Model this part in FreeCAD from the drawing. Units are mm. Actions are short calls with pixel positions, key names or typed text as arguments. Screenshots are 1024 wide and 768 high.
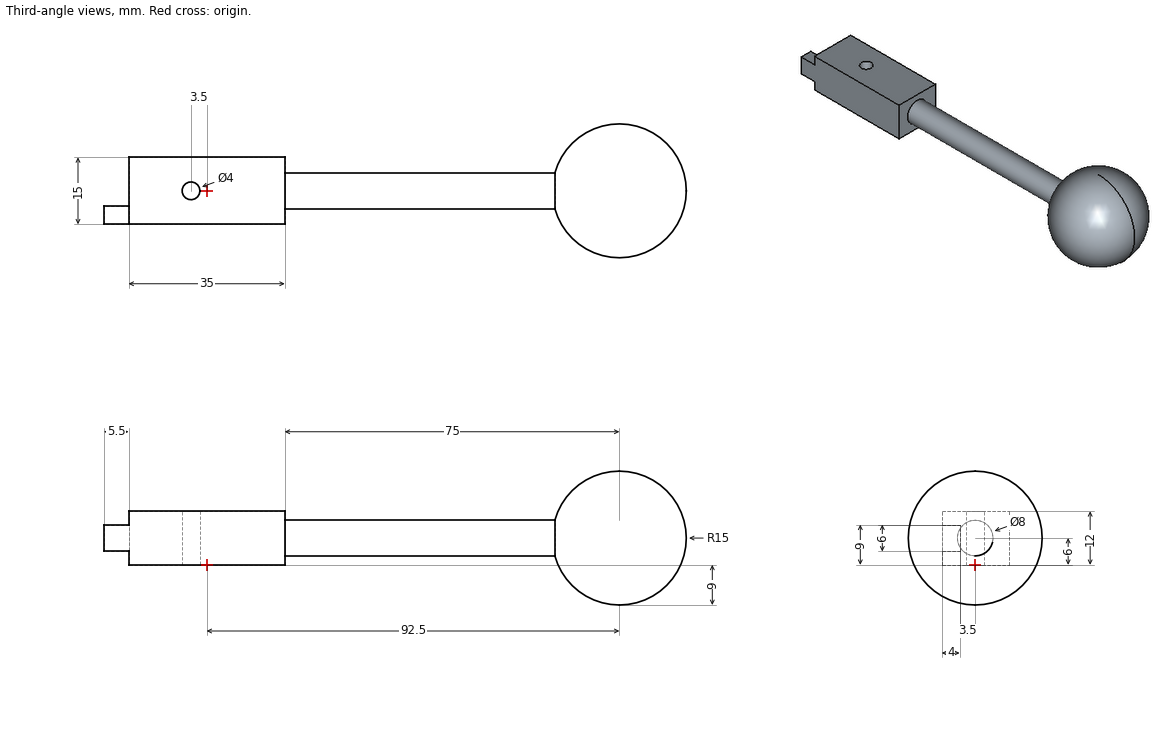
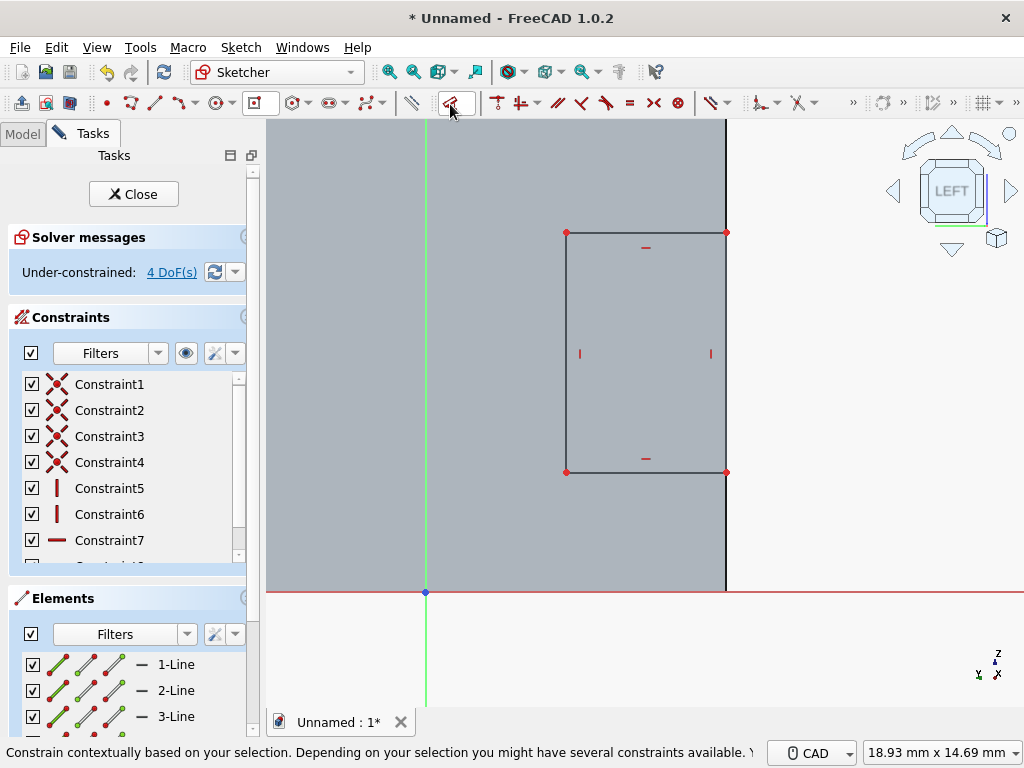
click(566, 305)
click(532, 353)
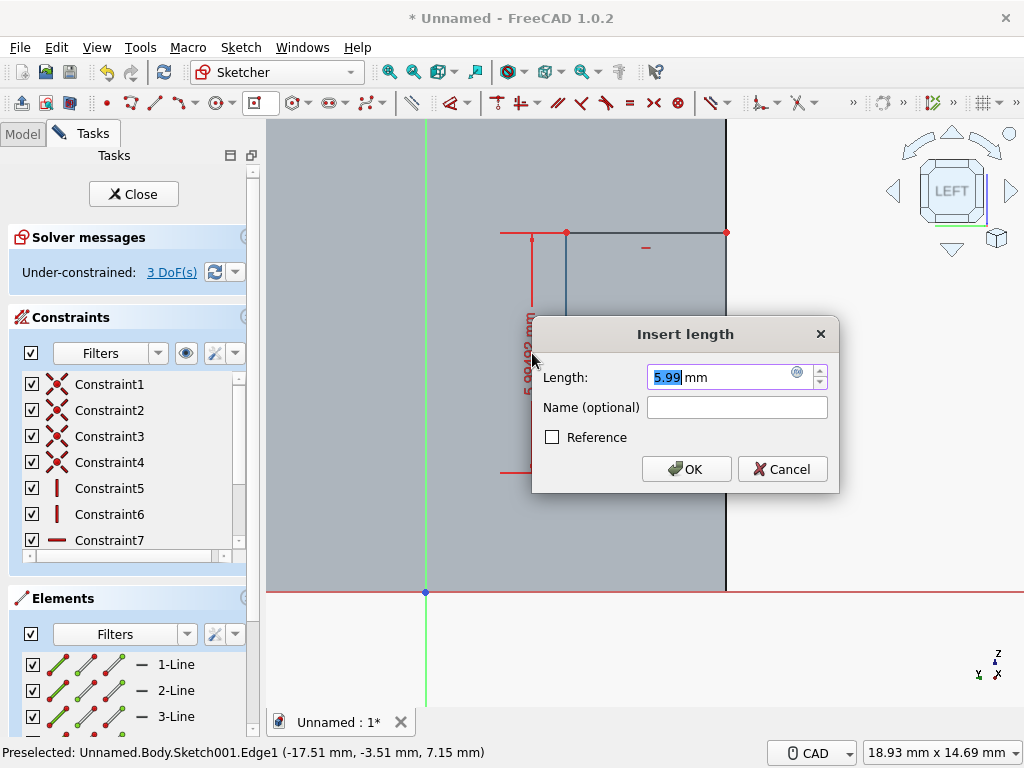
text(6)
key(Return)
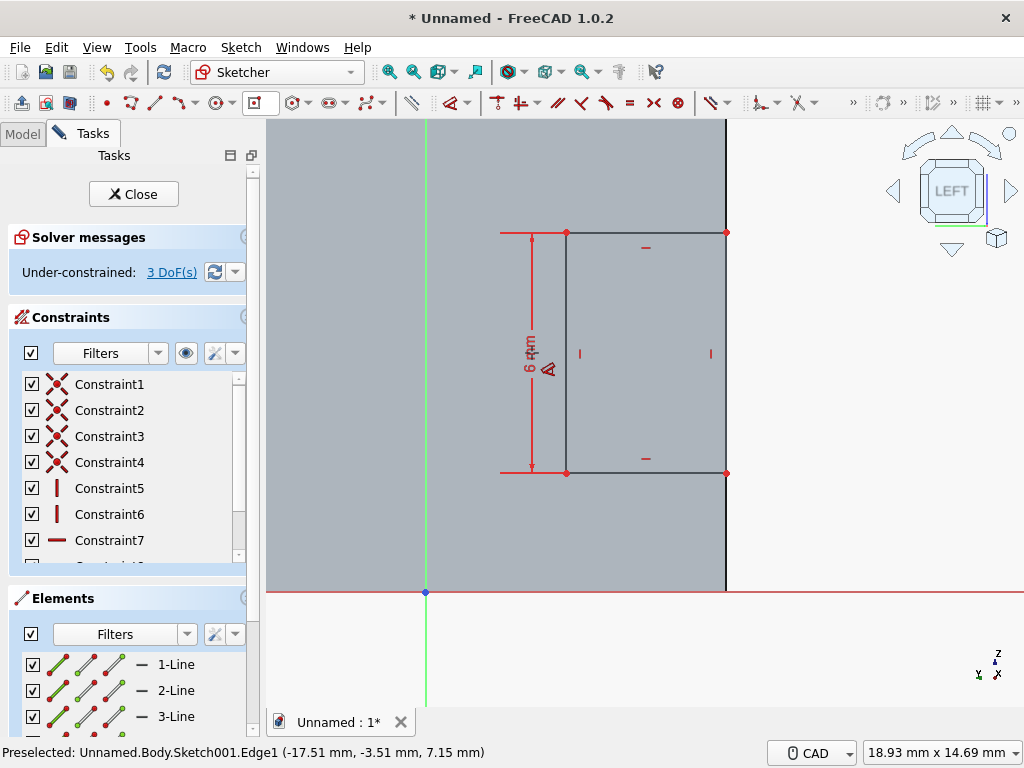
click(614, 473)
click(646, 507)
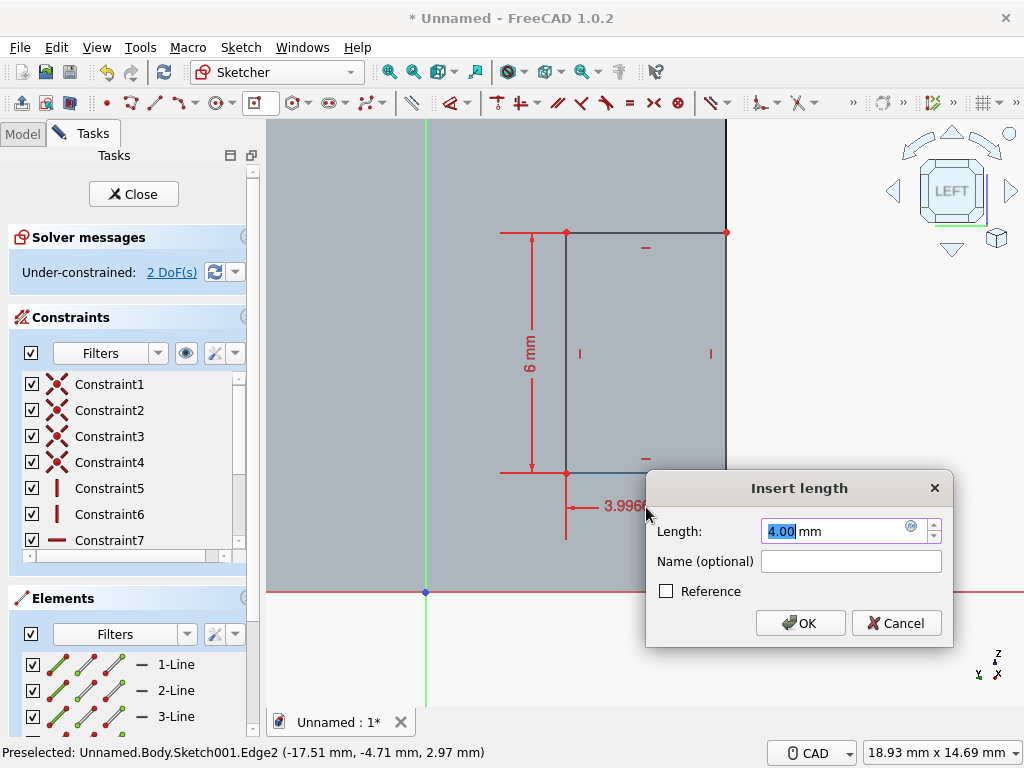
text(4)
key(Return)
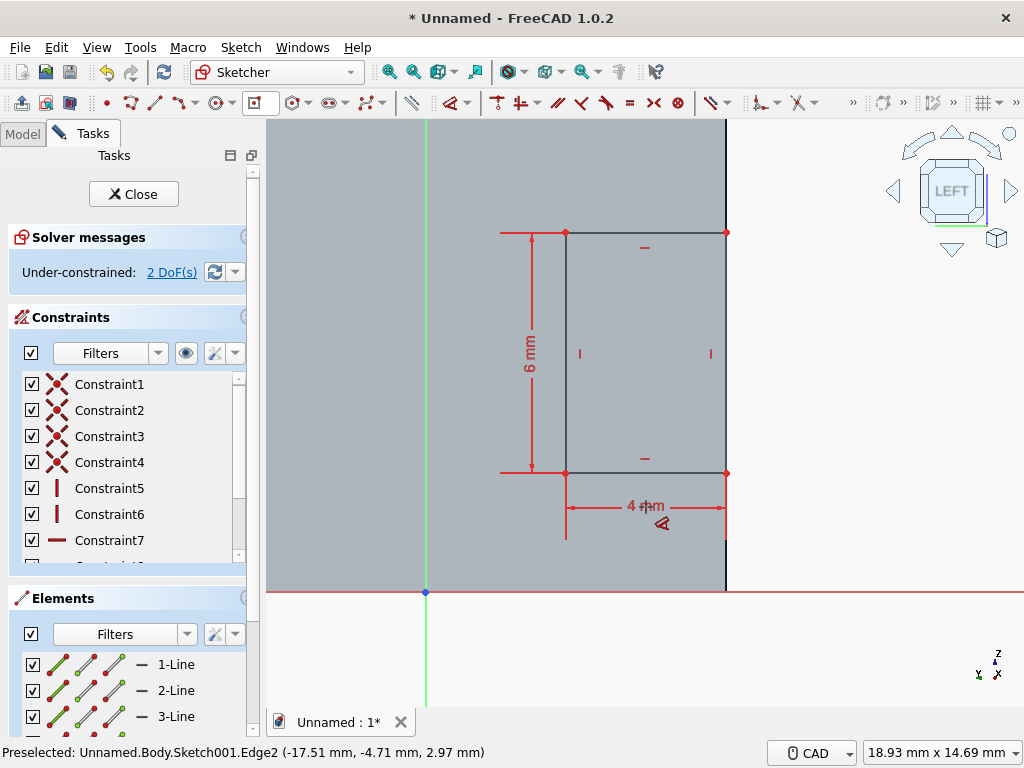
click(566, 233)
click(392, 413)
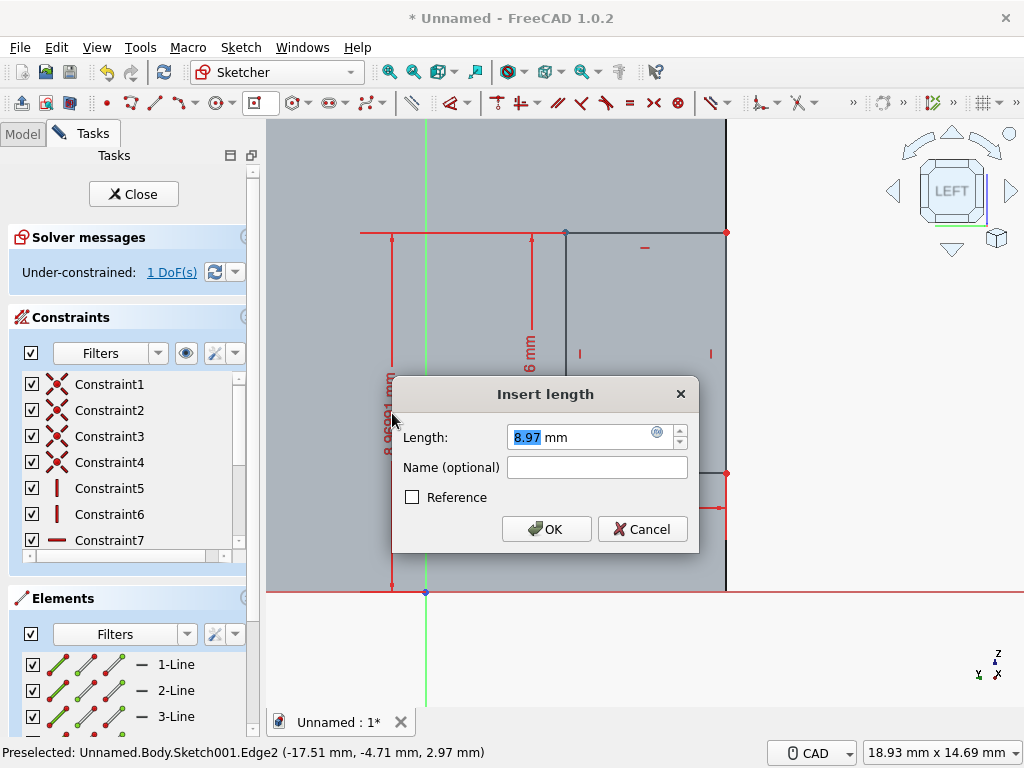
text(9)
key(Return)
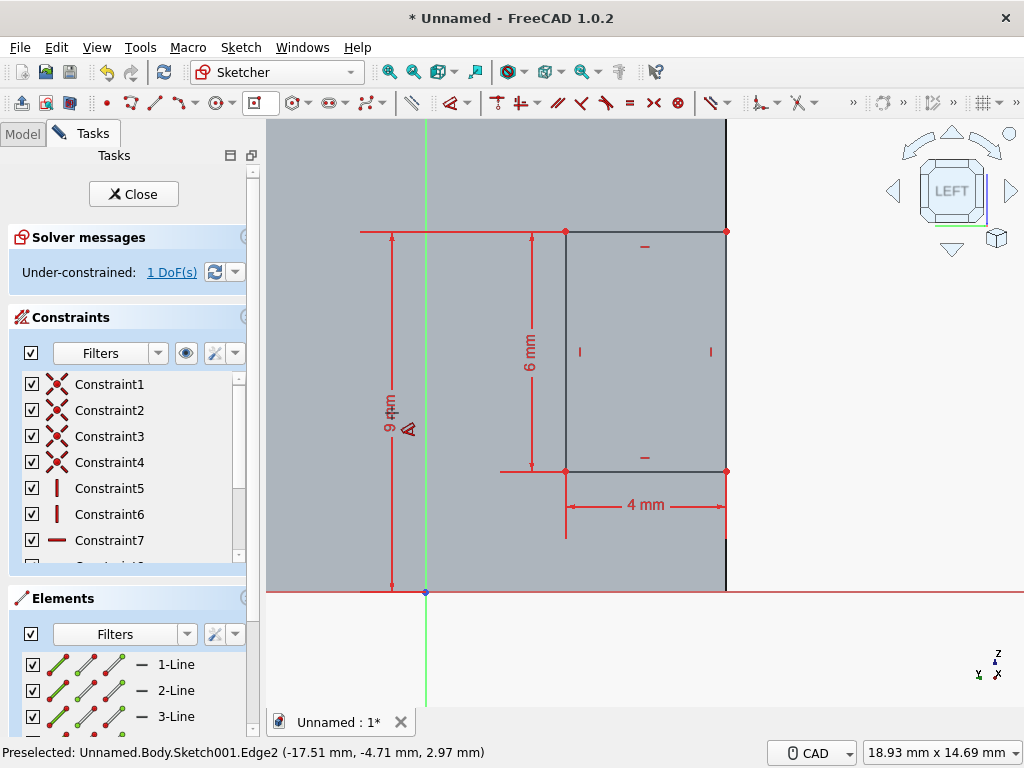
click(566, 232)
click(496, 626)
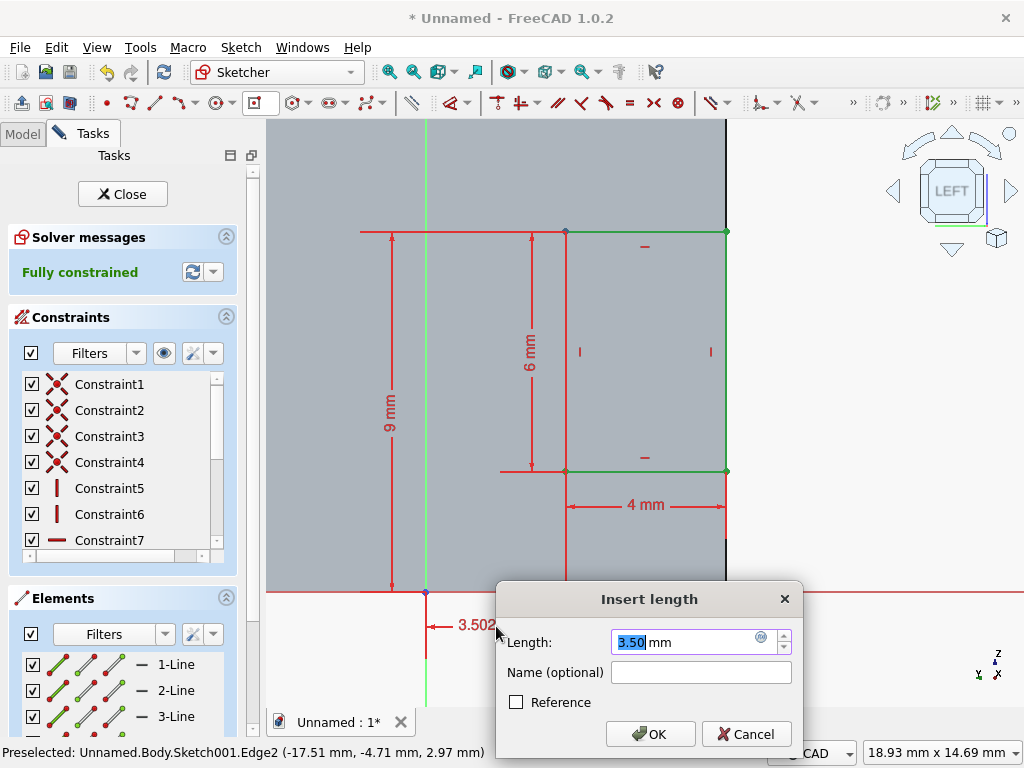
text(3.5)
key(Return)
key(Escape)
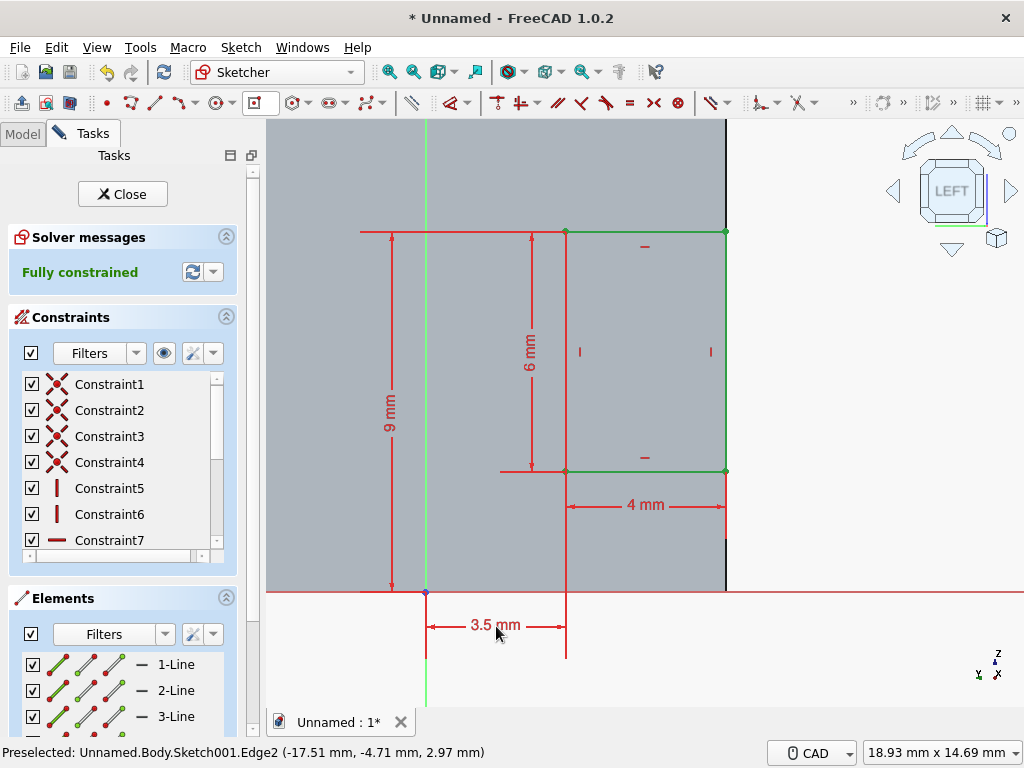
click(123, 194)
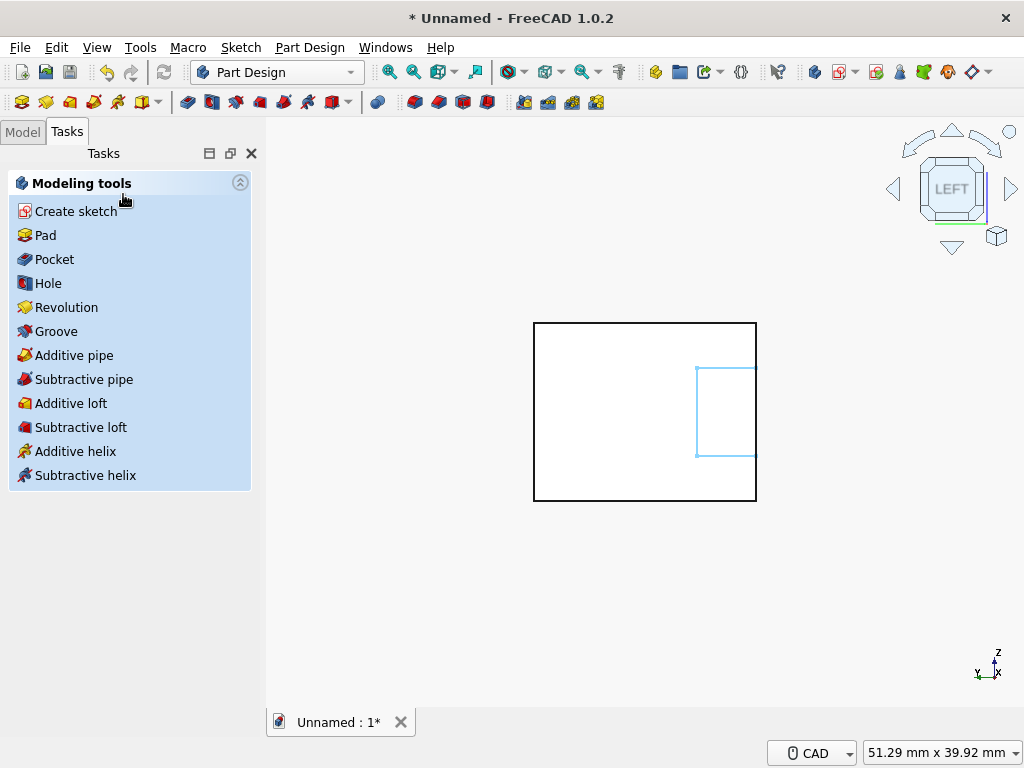
click(22, 102)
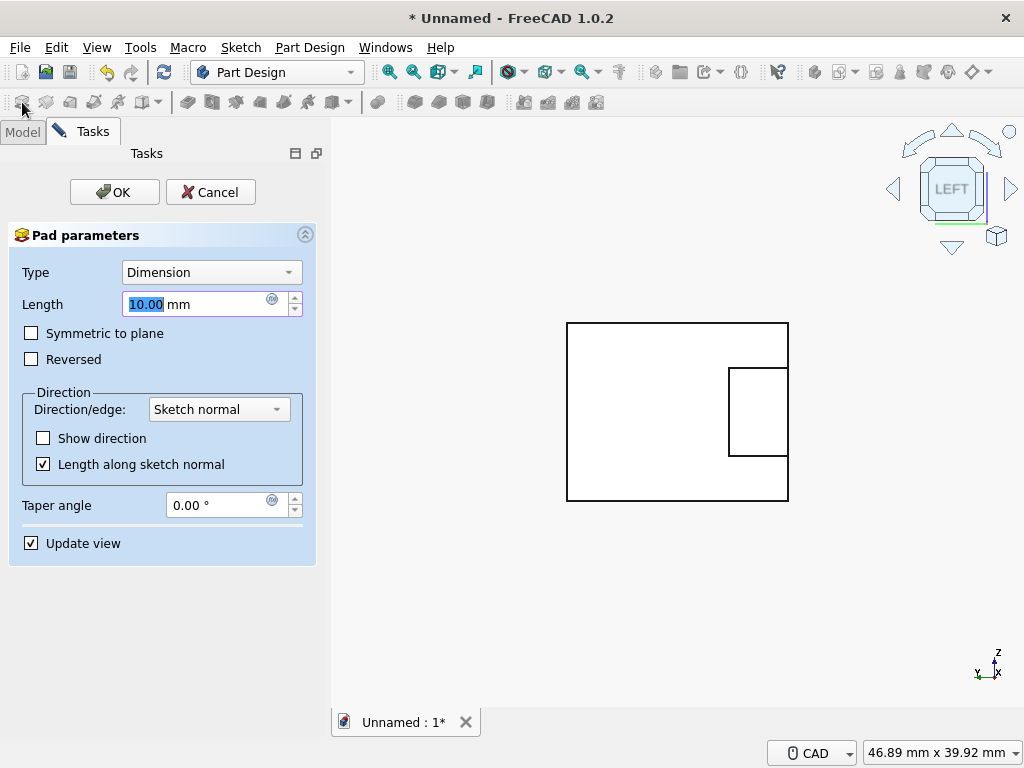
text(5.5)
key(Tab)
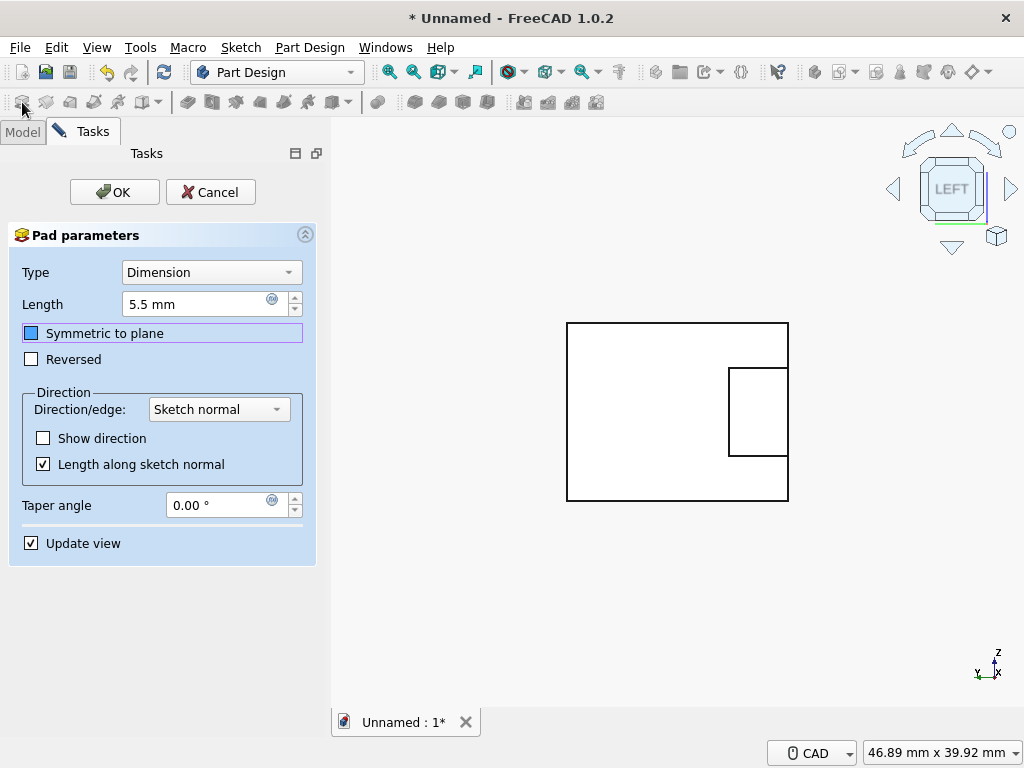
click(115, 192)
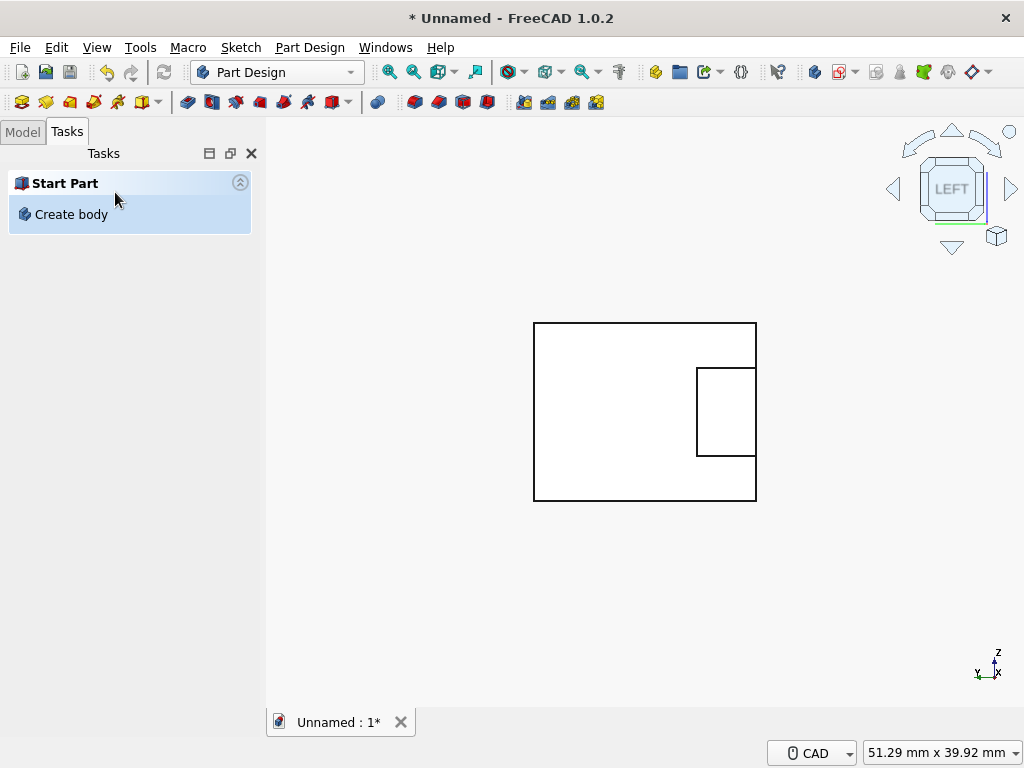
click(390, 72)